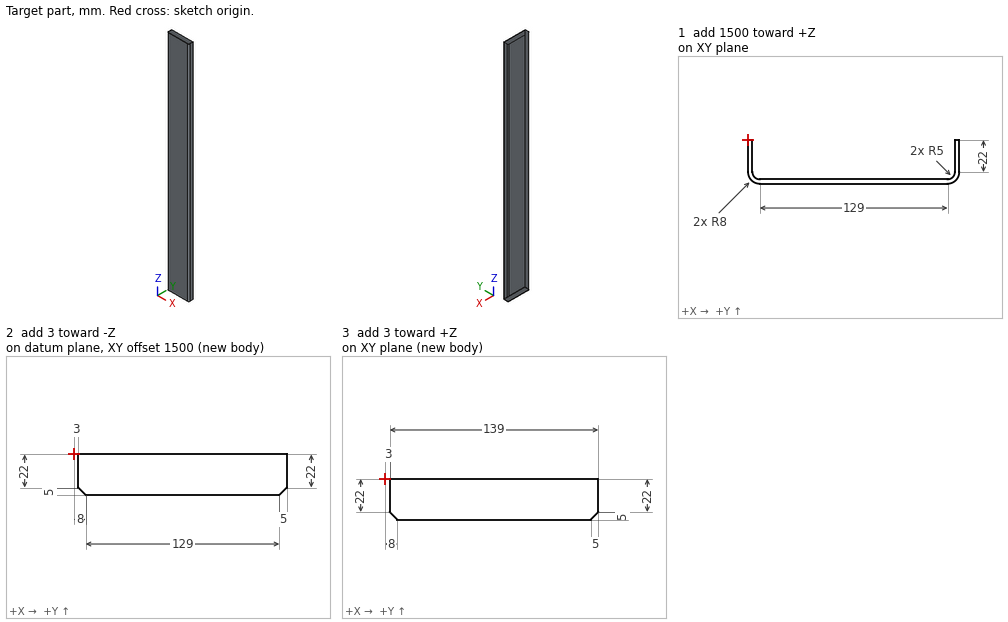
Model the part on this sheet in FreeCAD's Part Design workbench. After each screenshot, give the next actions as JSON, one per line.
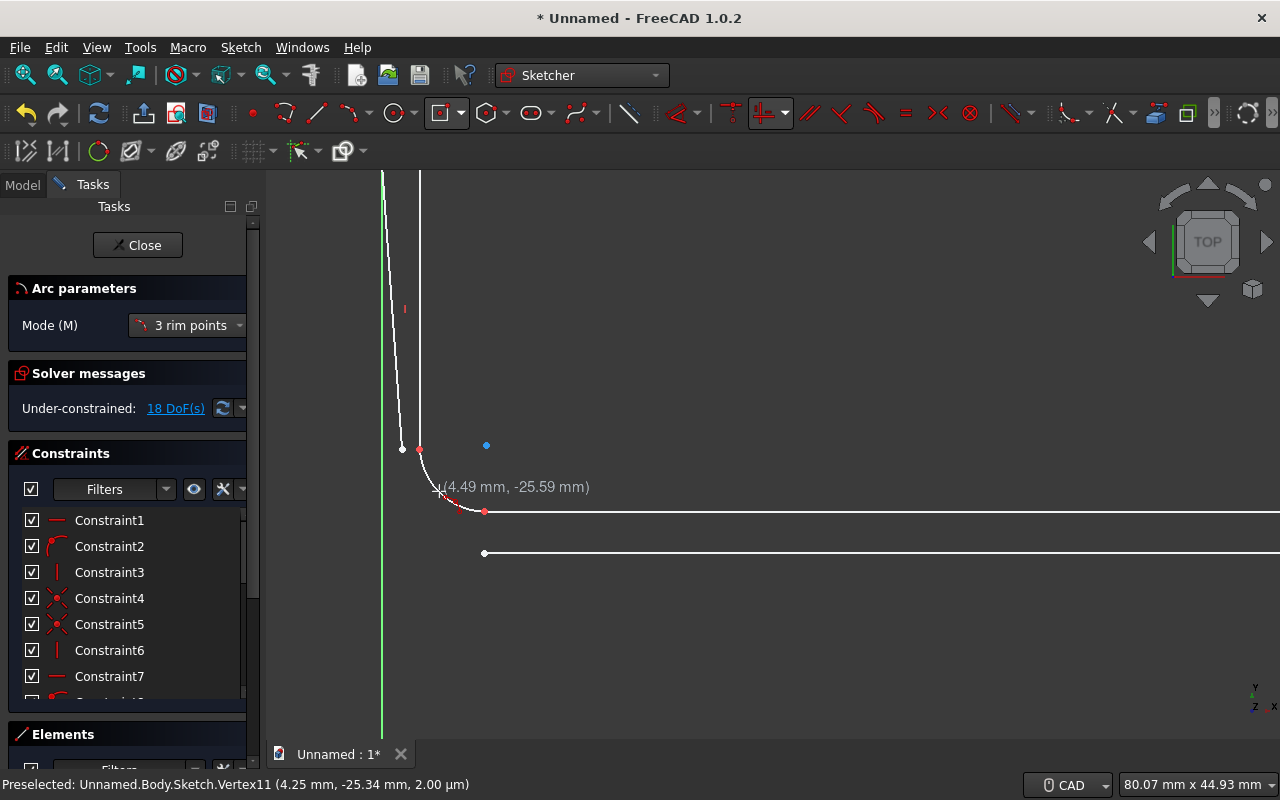
{"action": "left_click", "coordinate": [402, 449]}
{"action": "left_click", "coordinate": [484, 553]}
{"action": "left_click", "coordinate": [412, 518]}
{"action": "key", "text": "Escape"}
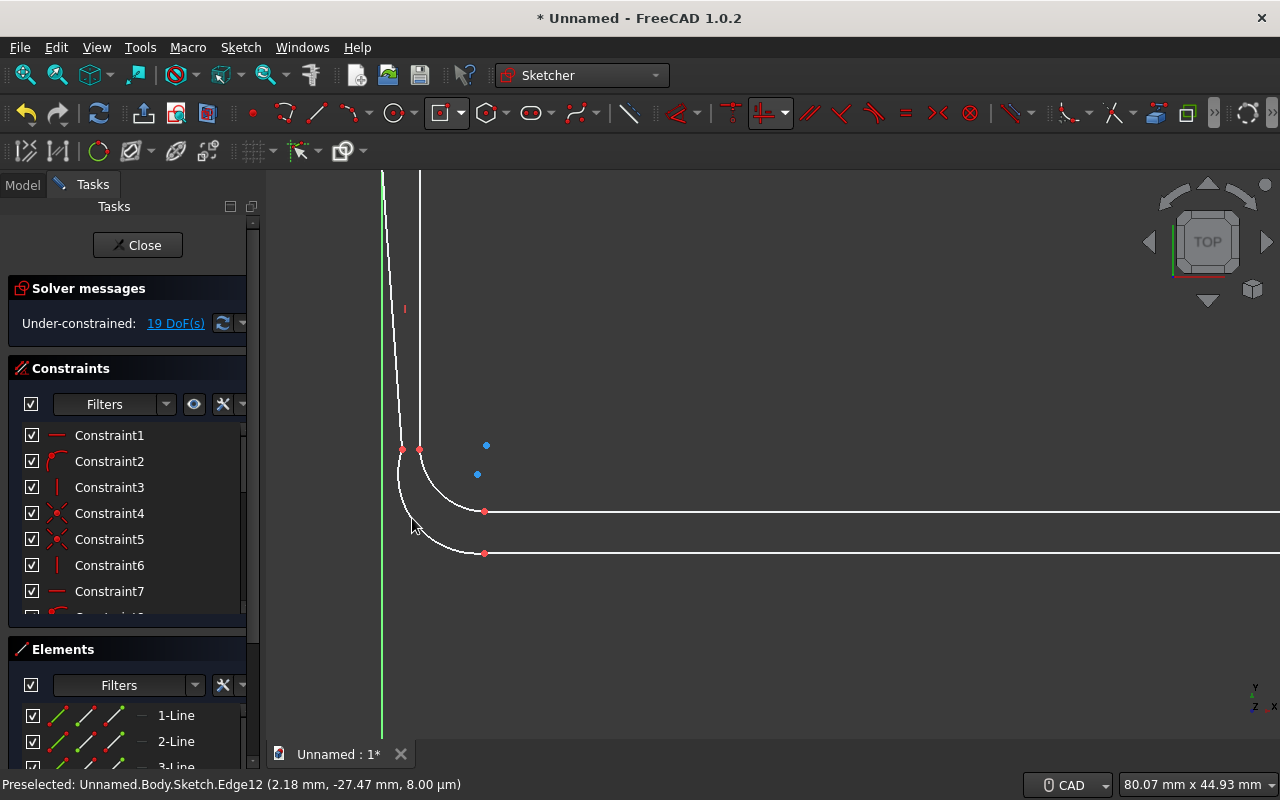
{"action": "scroll", "coordinate": [448, 496], "scroll_direction": "down", "scroll_amount": 6}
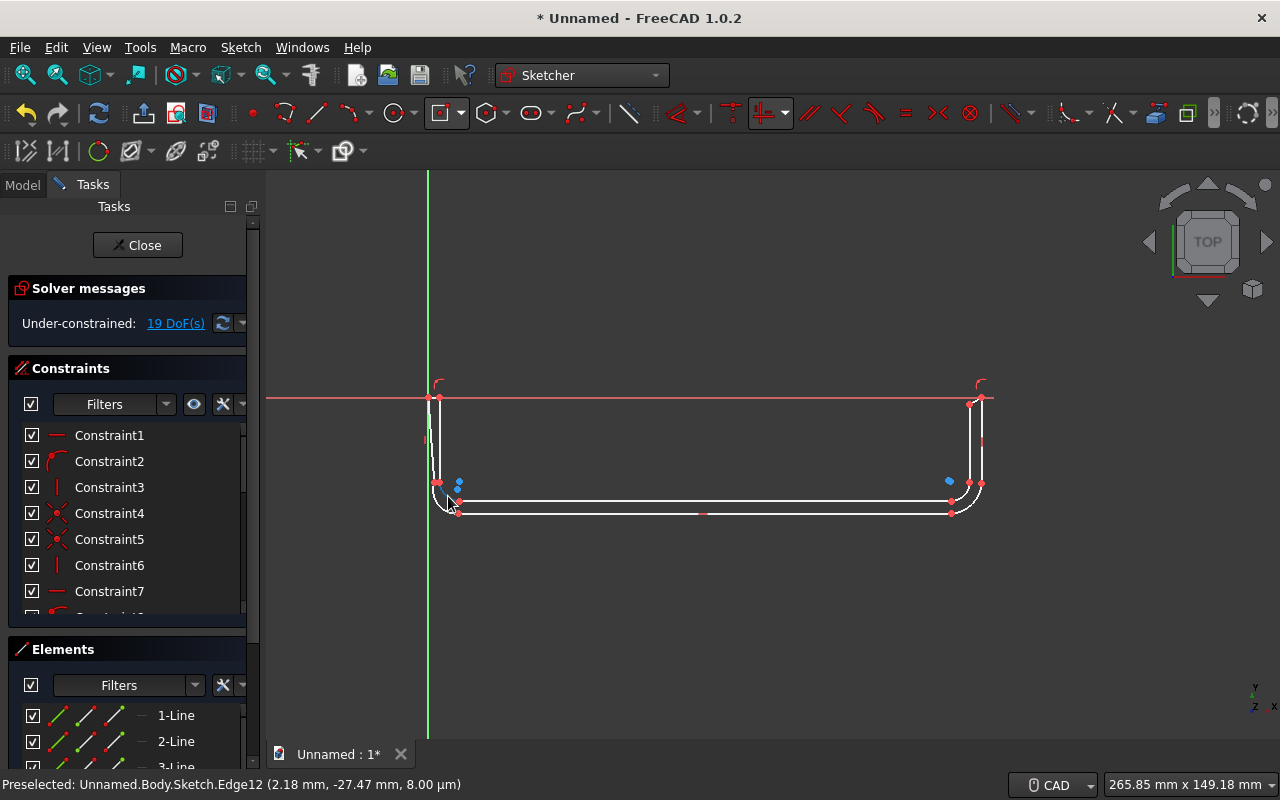
{"action": "left_click", "coordinate": [607, 514]}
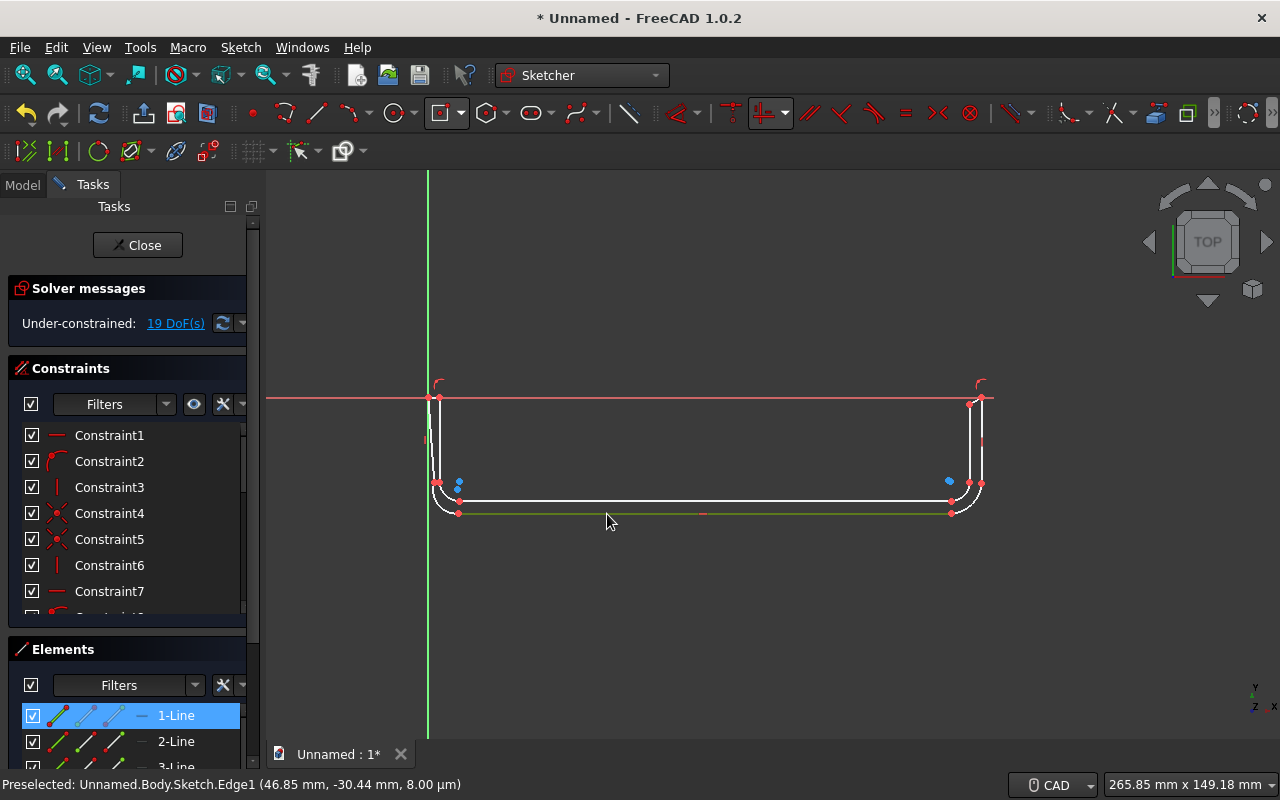
{"action": "left_click", "coordinate": [965, 510]}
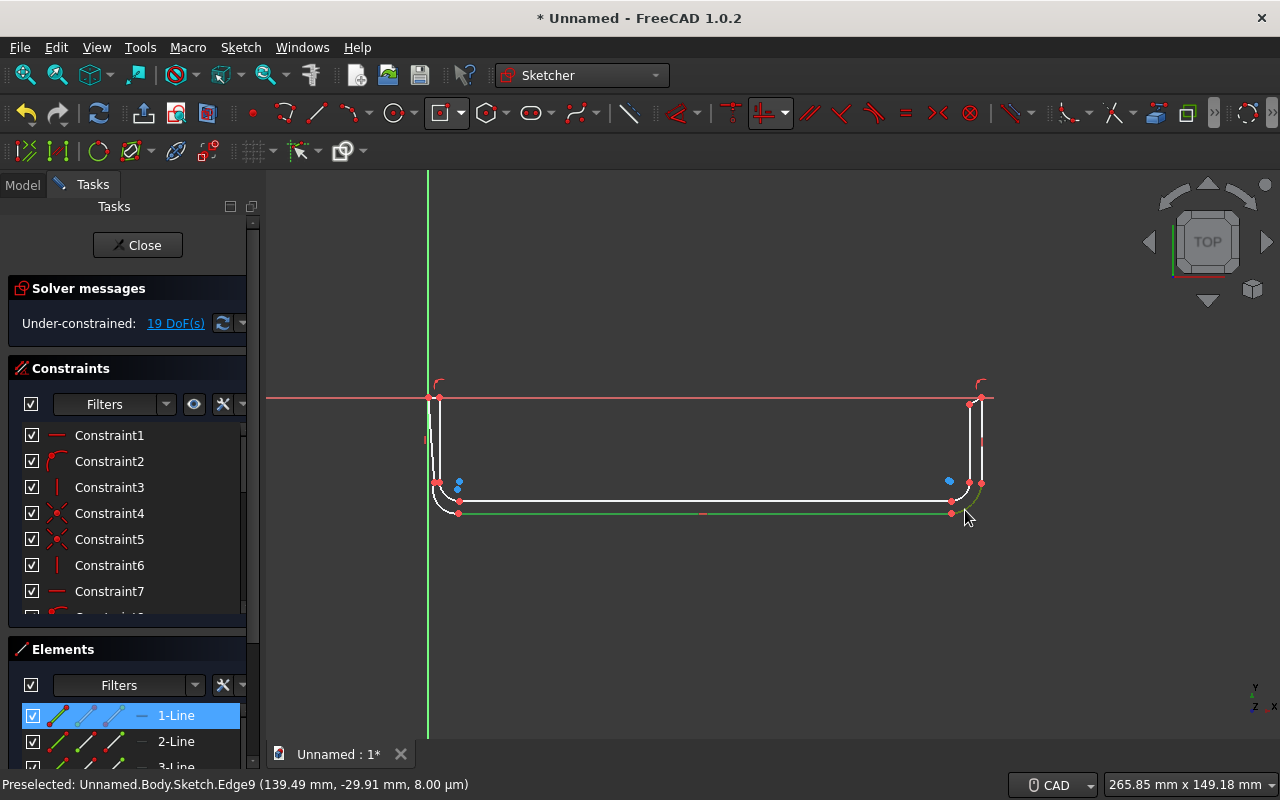
{"action": "key", "text": "t"}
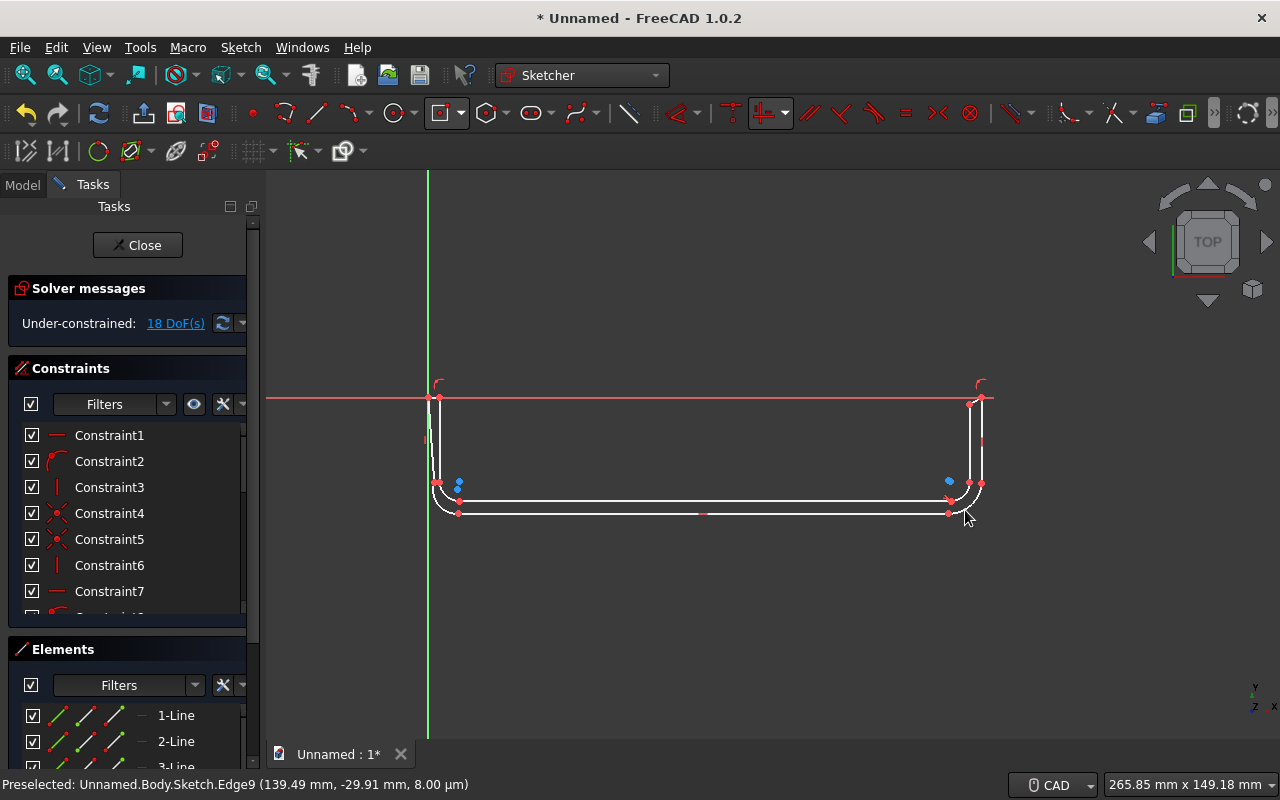
{"action": "left_click", "coordinate": [606, 514]}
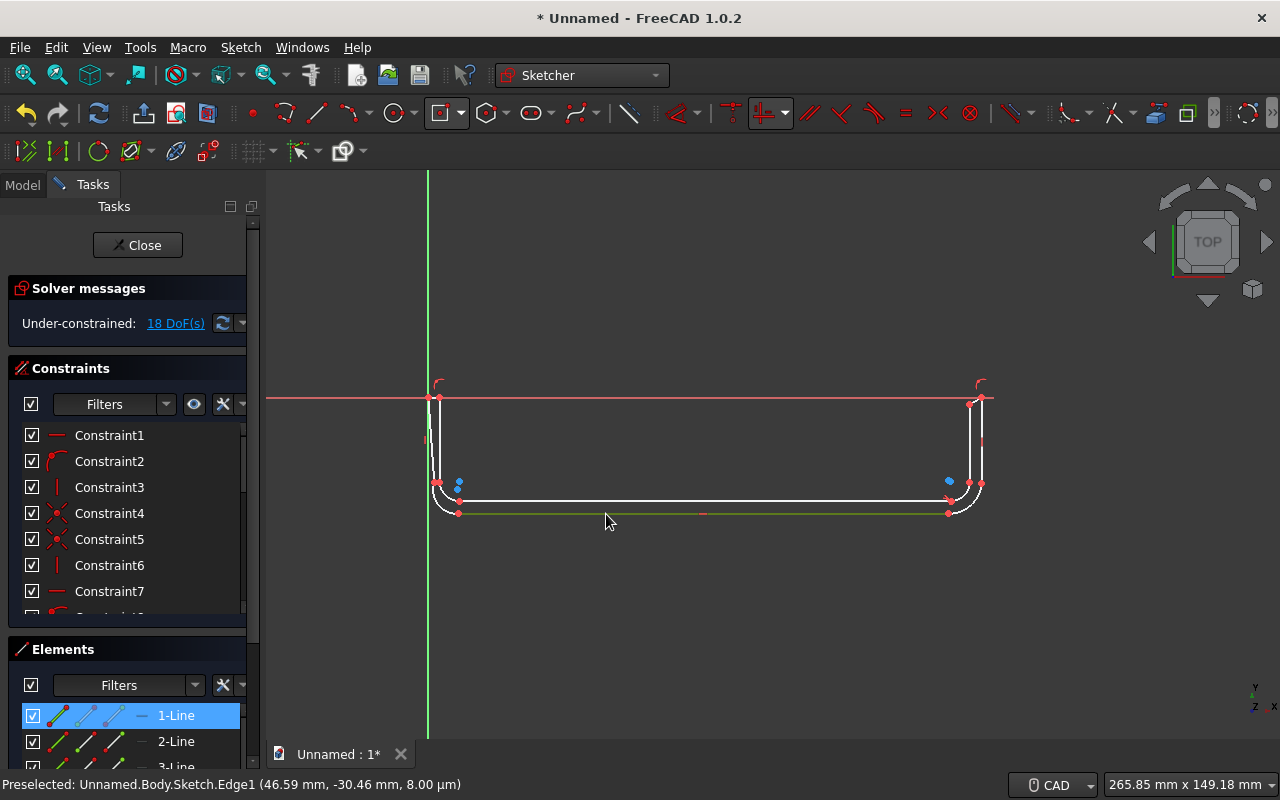
{"action": "left_click", "coordinate": [445, 511]}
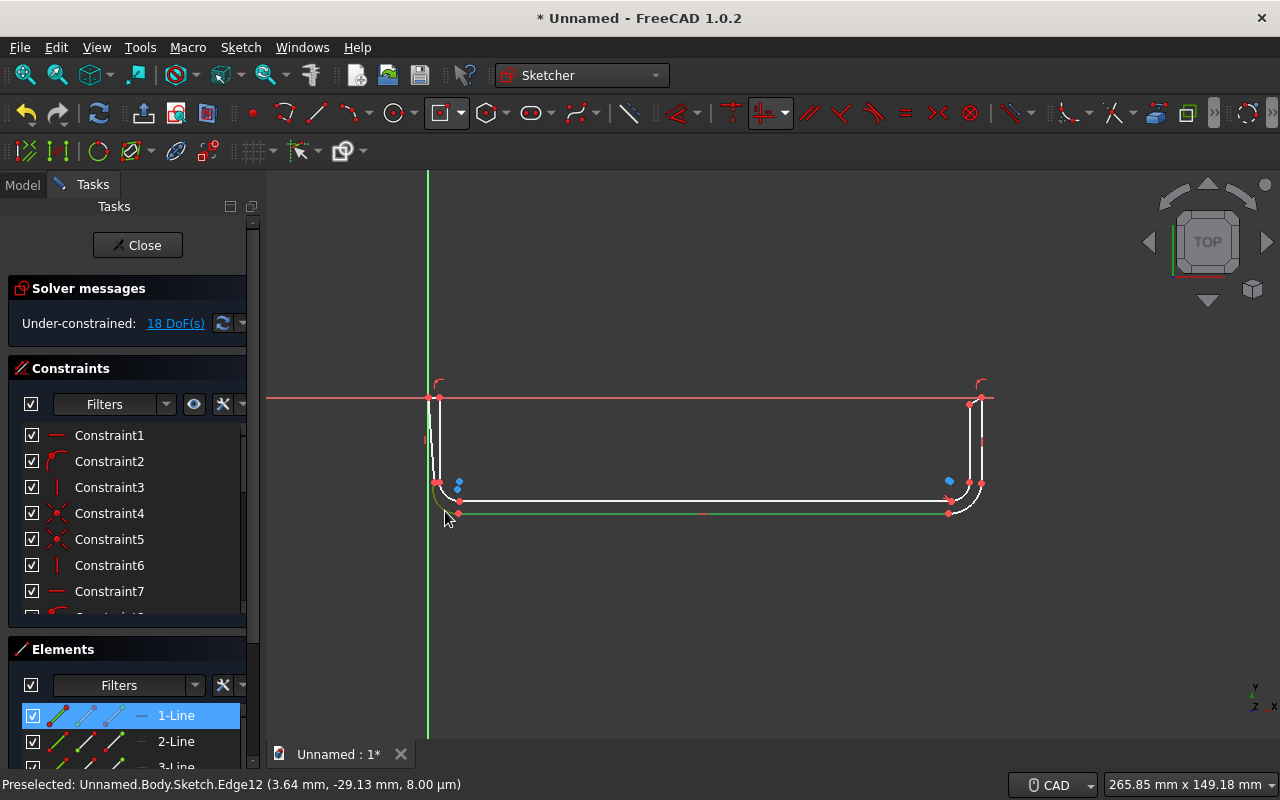
{"action": "left_click", "coordinate": [874, 114]}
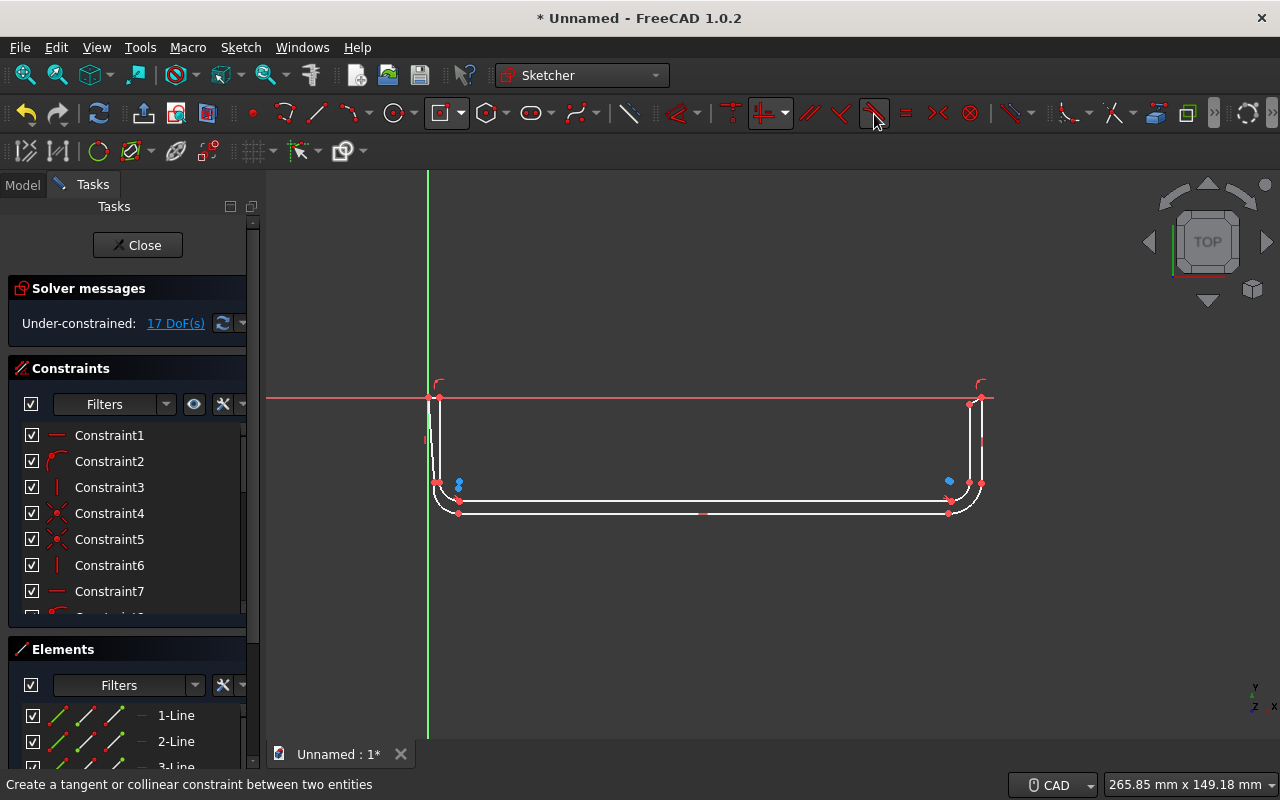
{"action": "left_click", "coordinate": [982, 457]}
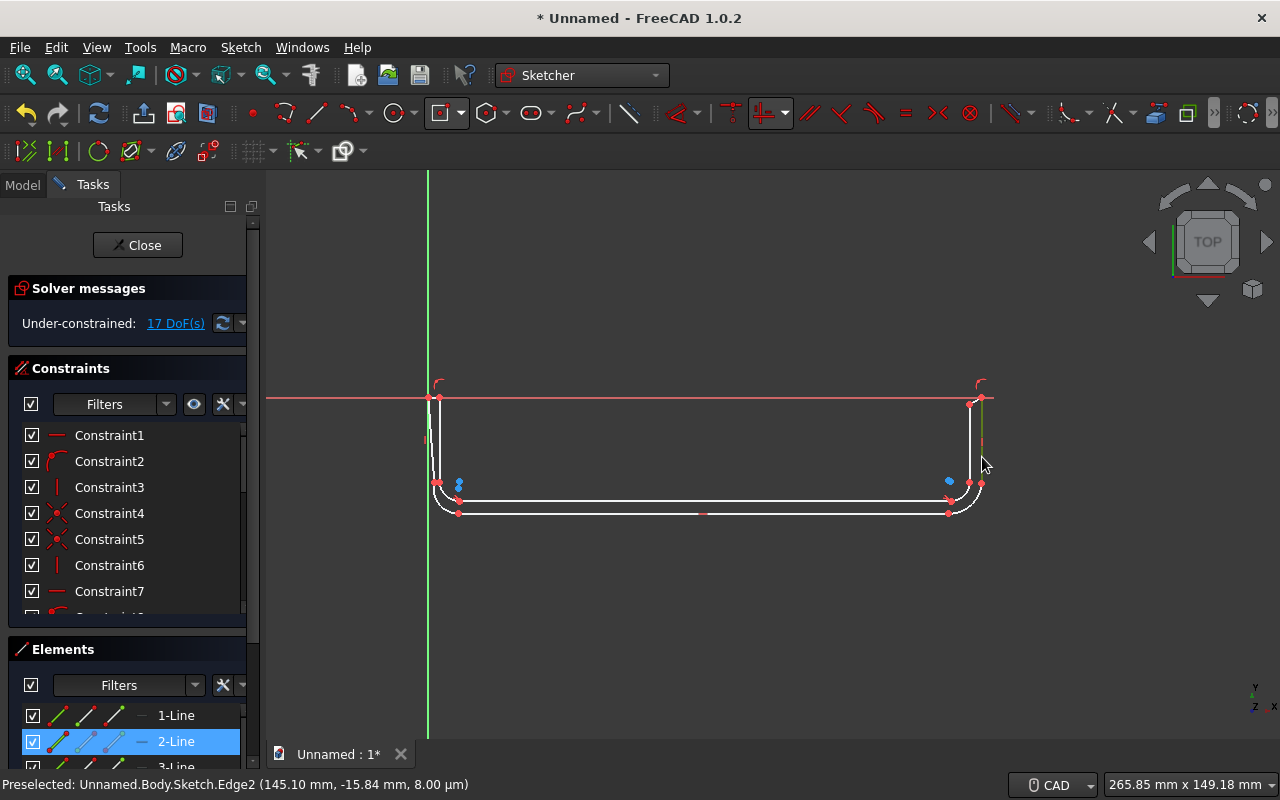
{"action": "left_click", "coordinate": [963, 510]}